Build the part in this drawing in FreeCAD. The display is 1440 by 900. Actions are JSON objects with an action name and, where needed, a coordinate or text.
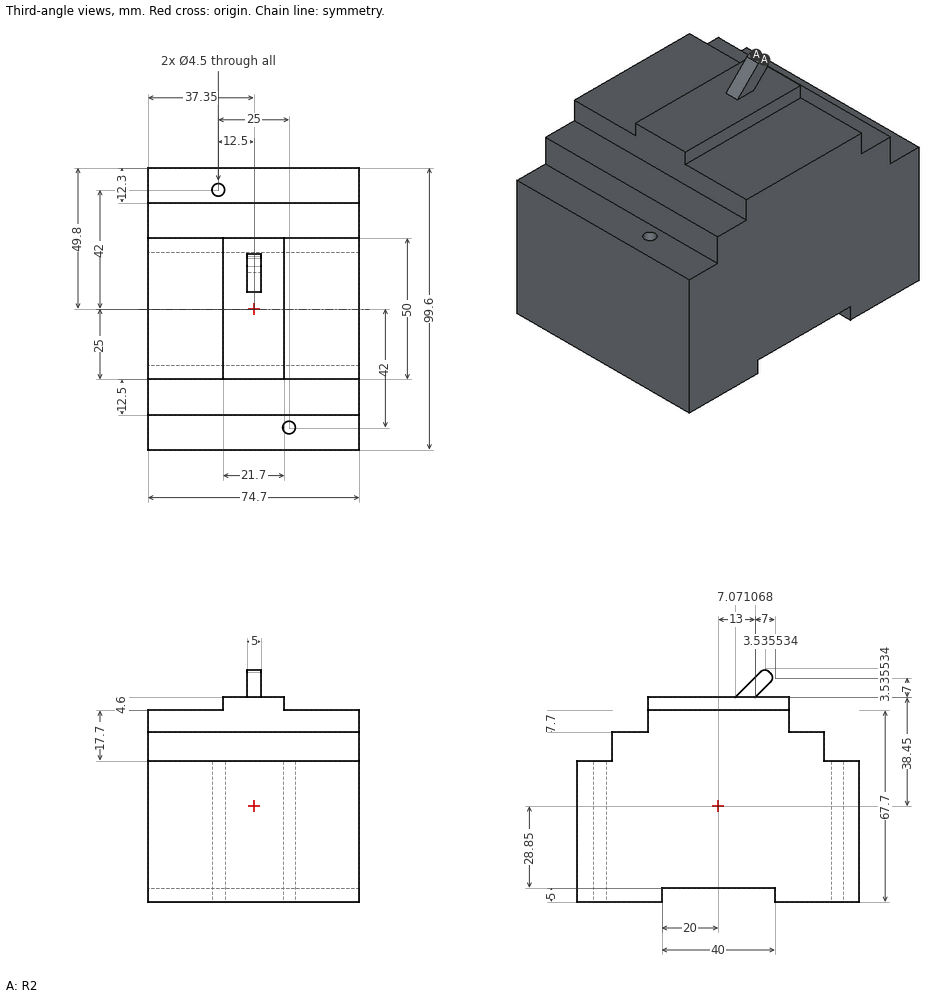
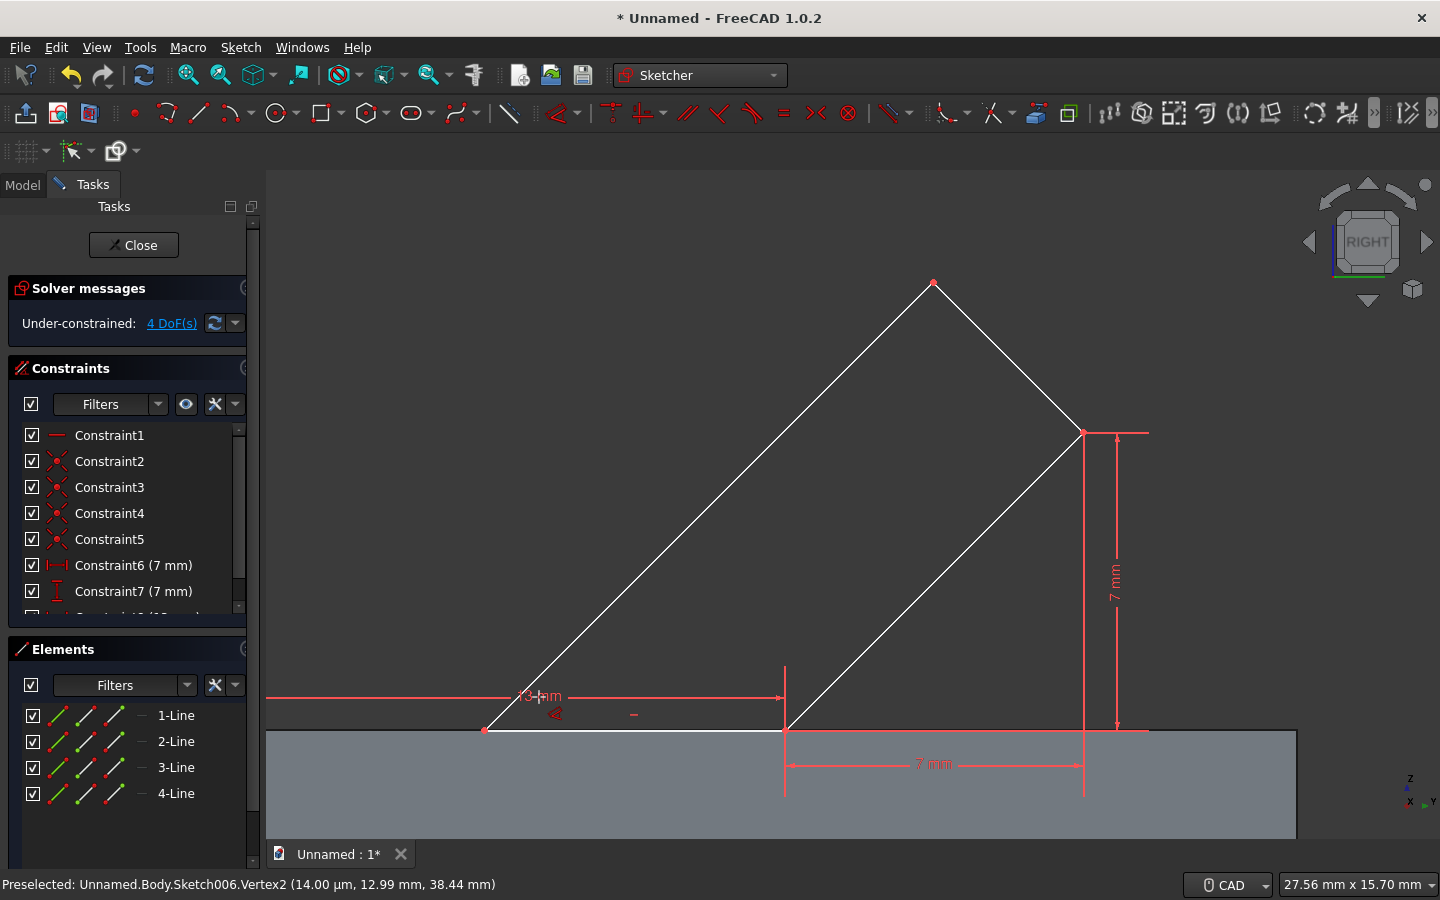
{"action": "left_click", "coordinate": [484, 731]}
{"action": "left_click", "coordinate": [518, 771]}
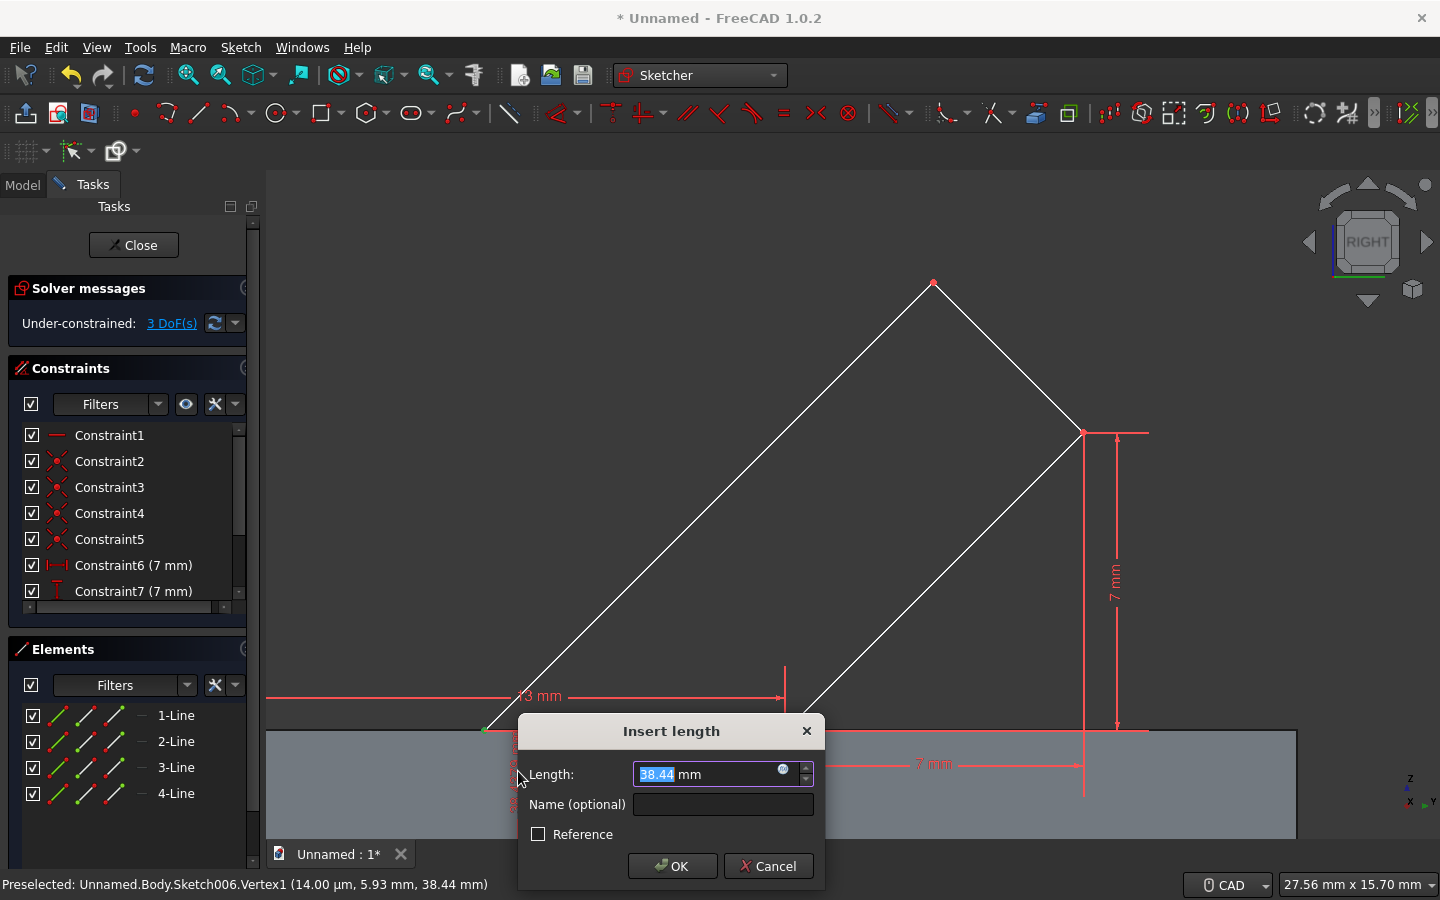
{"action": "type", "text": "38.45"}
{"action": "key", "text": "Return"}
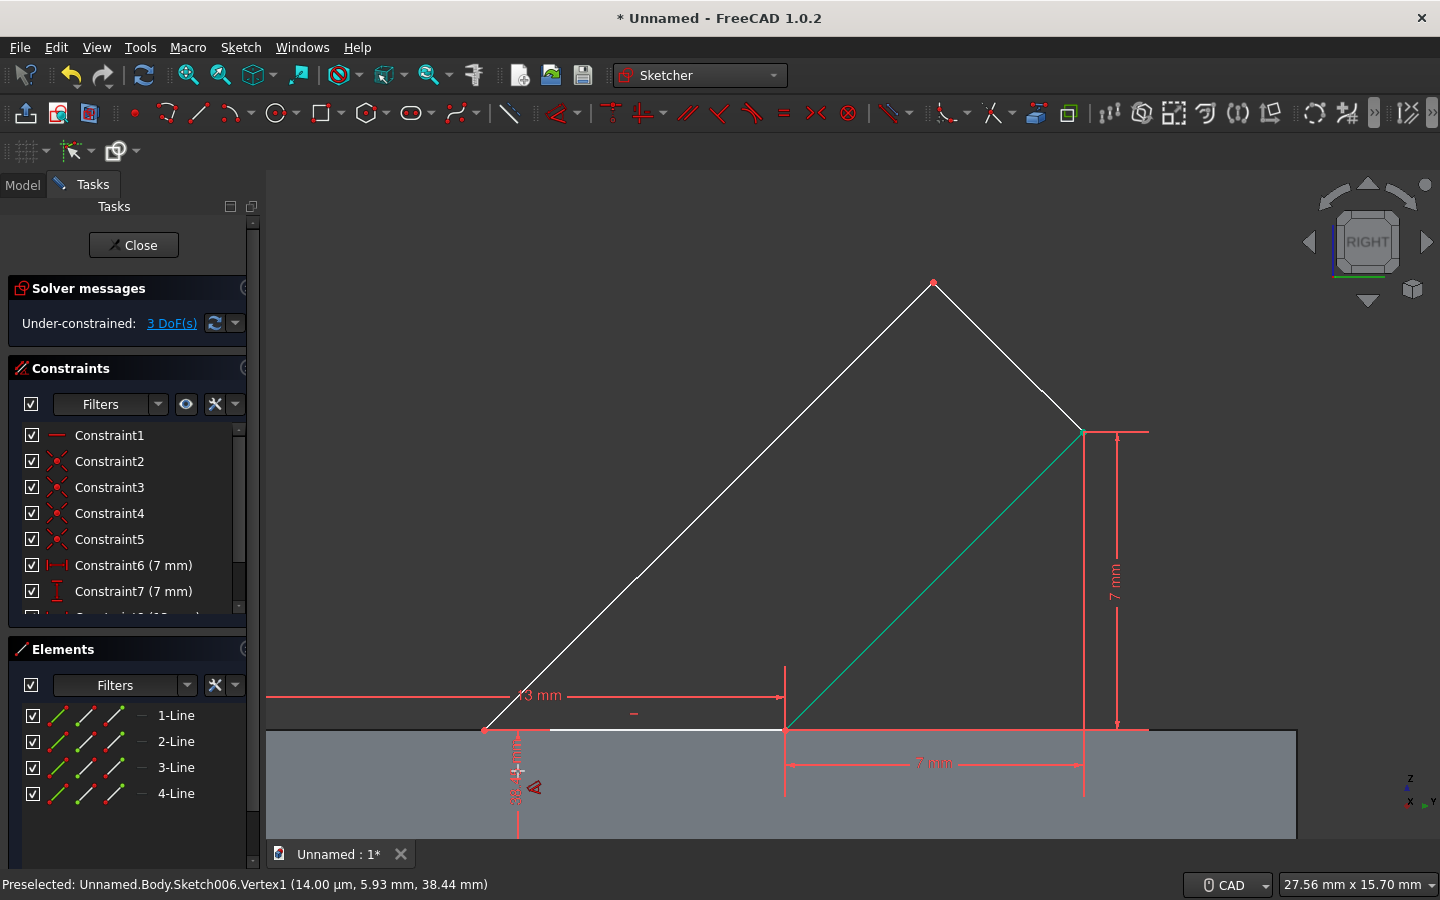
{"action": "left_click", "coordinate": [574, 730]}
{"action": "left_click", "coordinate": [635, 764]}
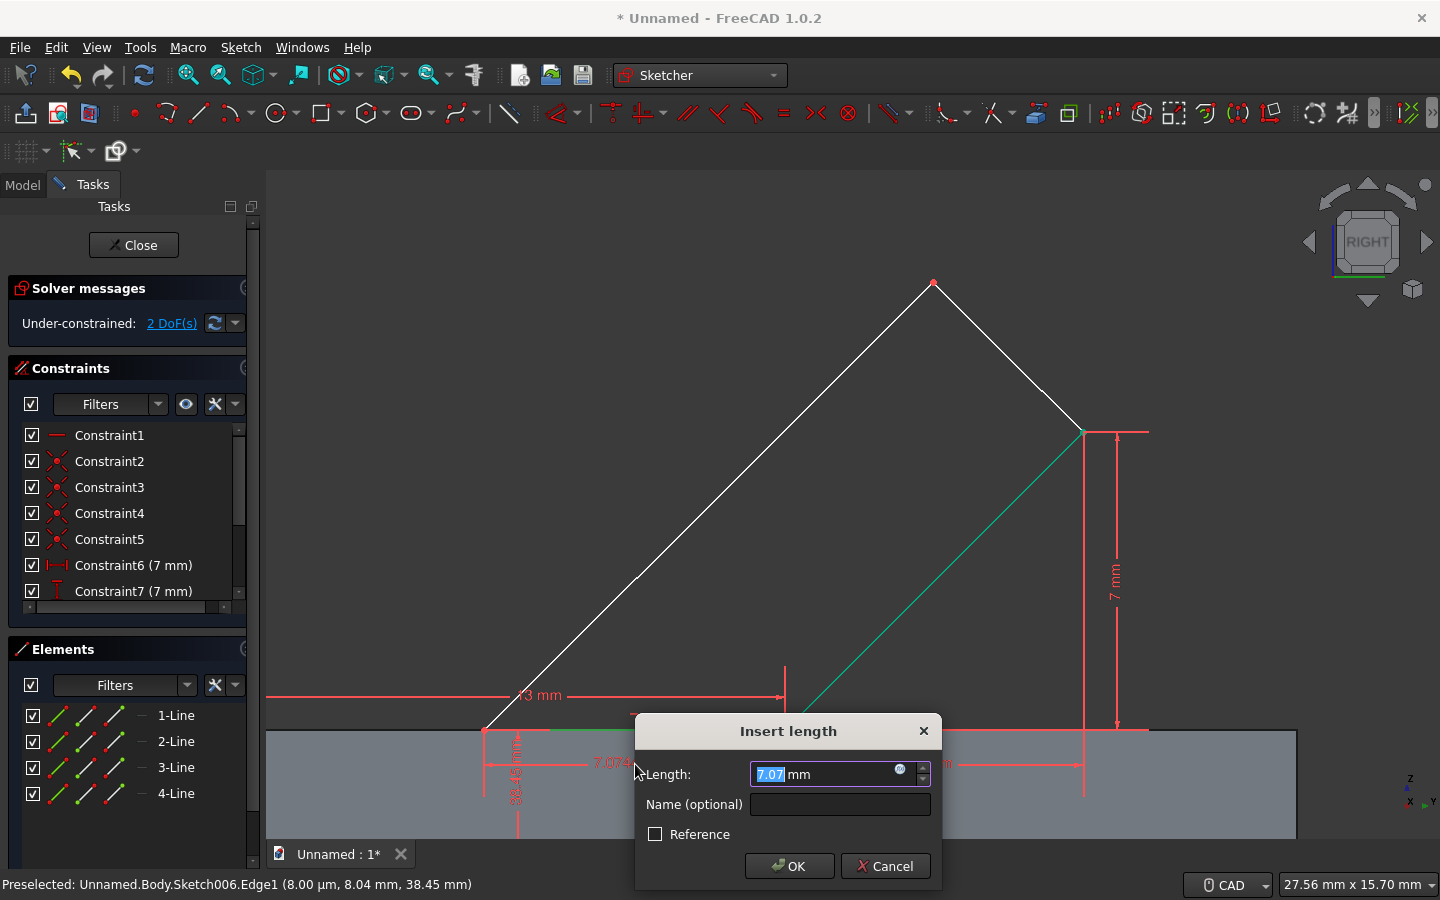
{"action": "type", "text": "7.071068"}
{"action": "key", "text": "Return"}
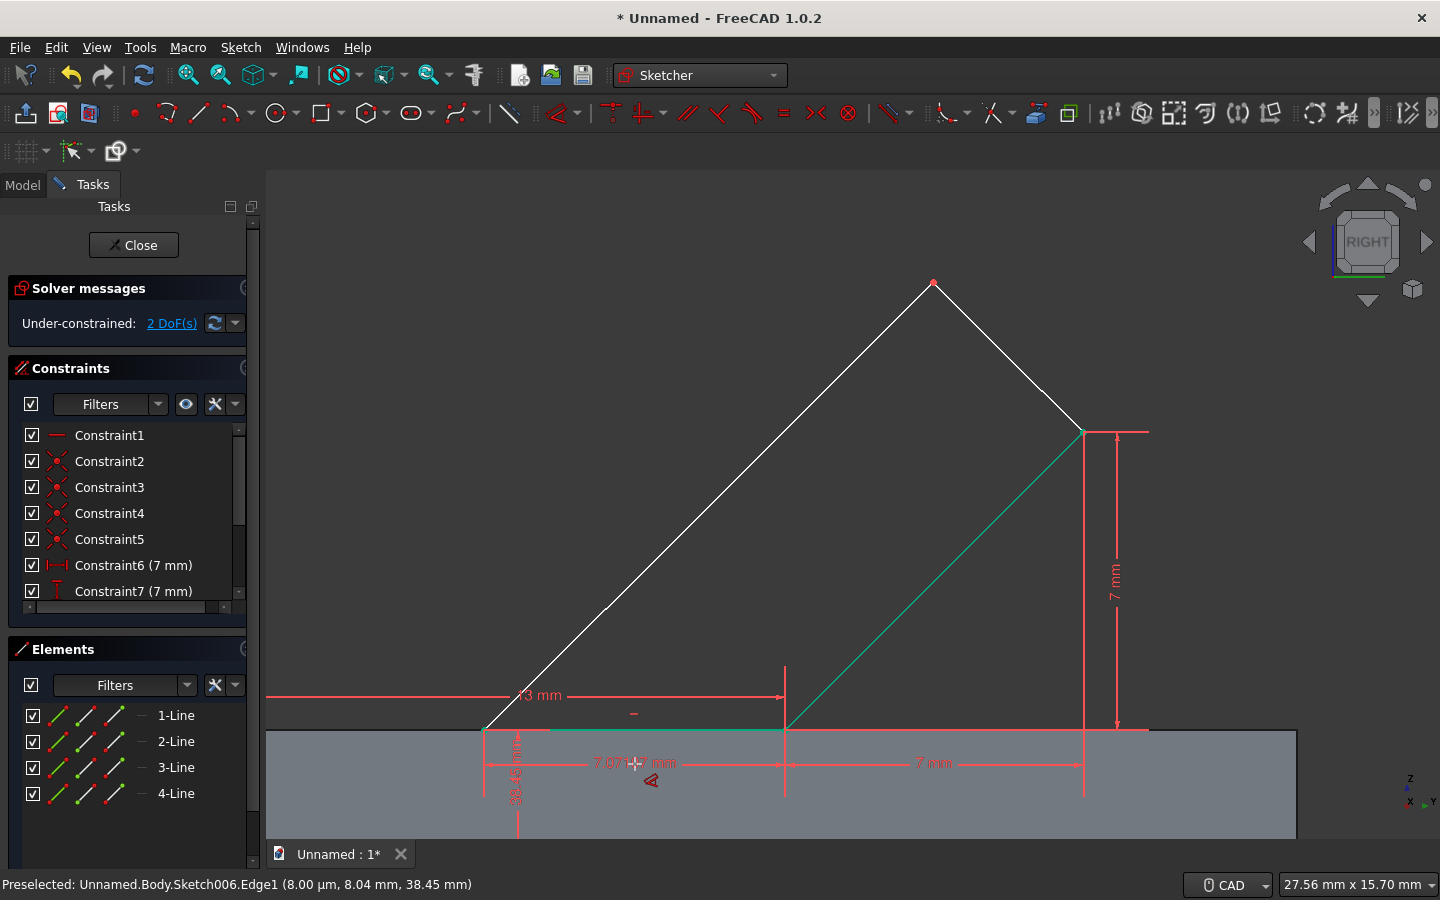
{"action": "left_click", "coordinate": [1038, 387]}
{"action": "left_click", "coordinate": [1008, 249]}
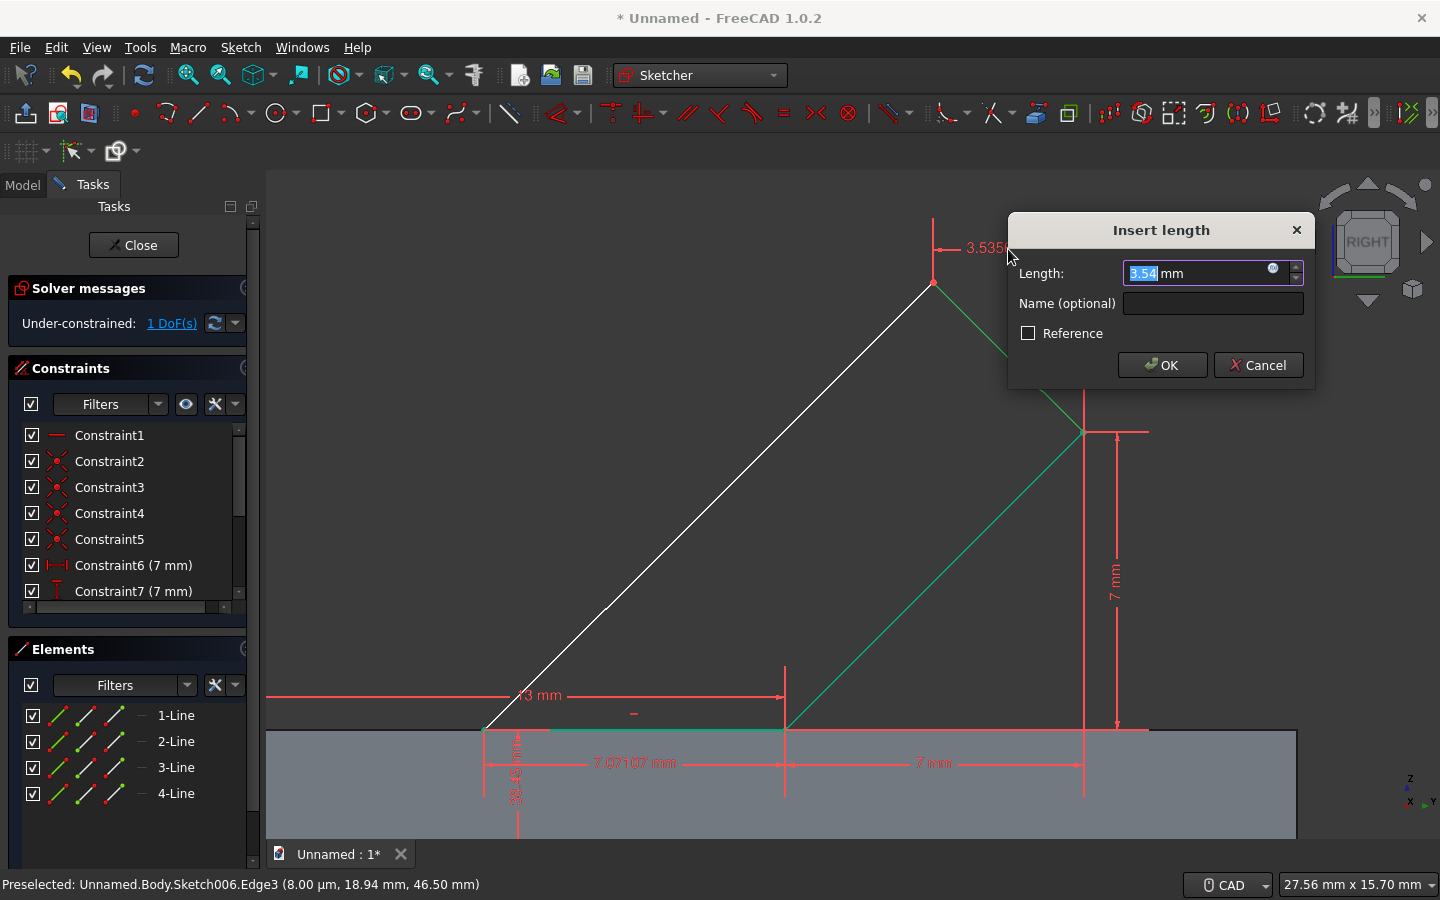
{"action": "type", "text": "3.535534"}
{"action": "key", "text": "Return"}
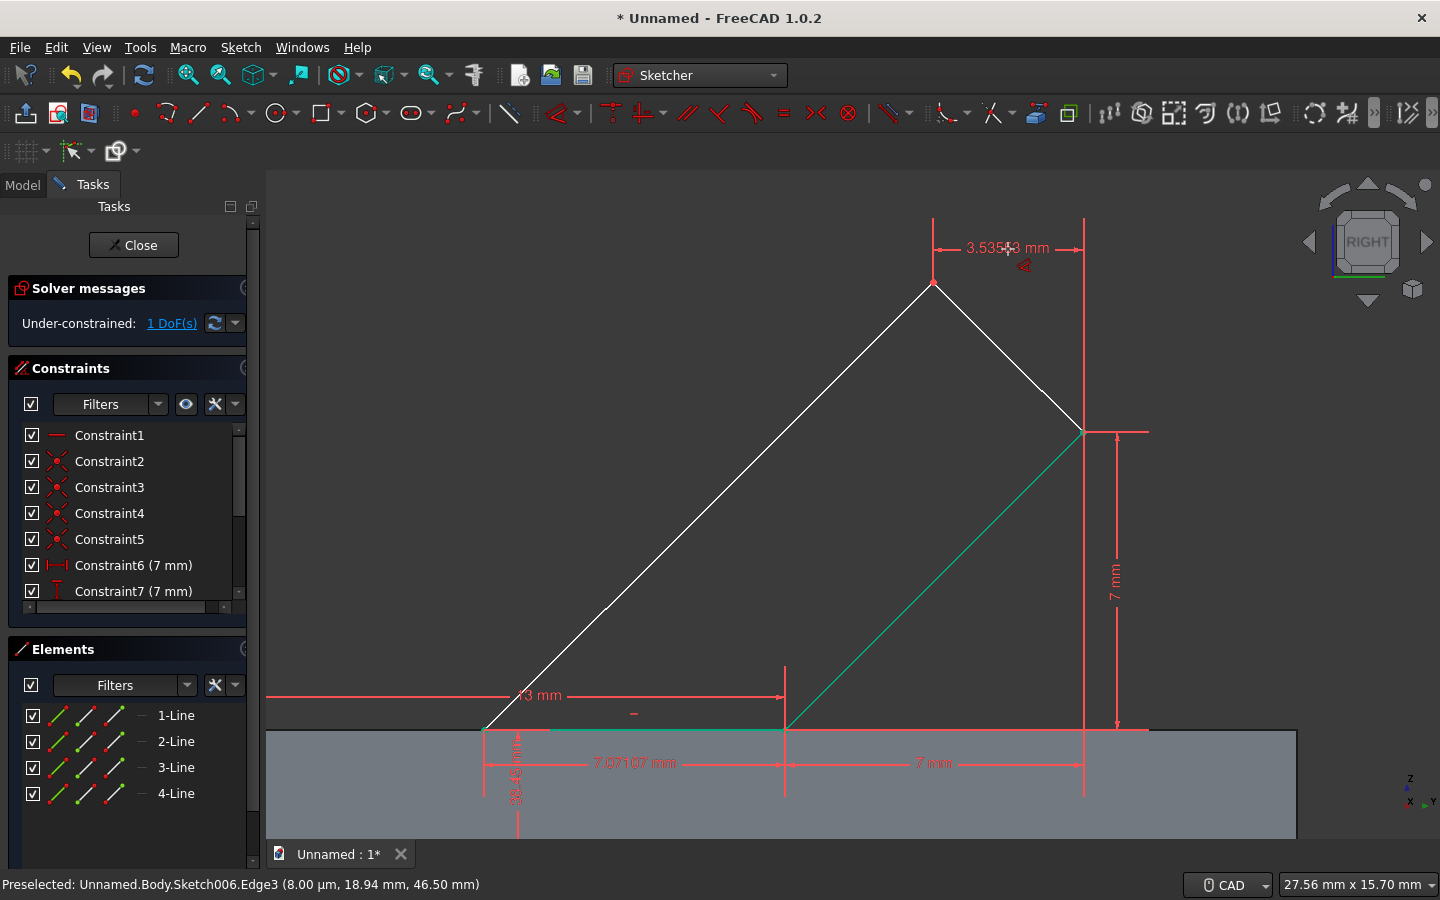
{"action": "left_click", "coordinate": [1038, 387]}
{"action": "left_click", "coordinate": [1118, 358]}